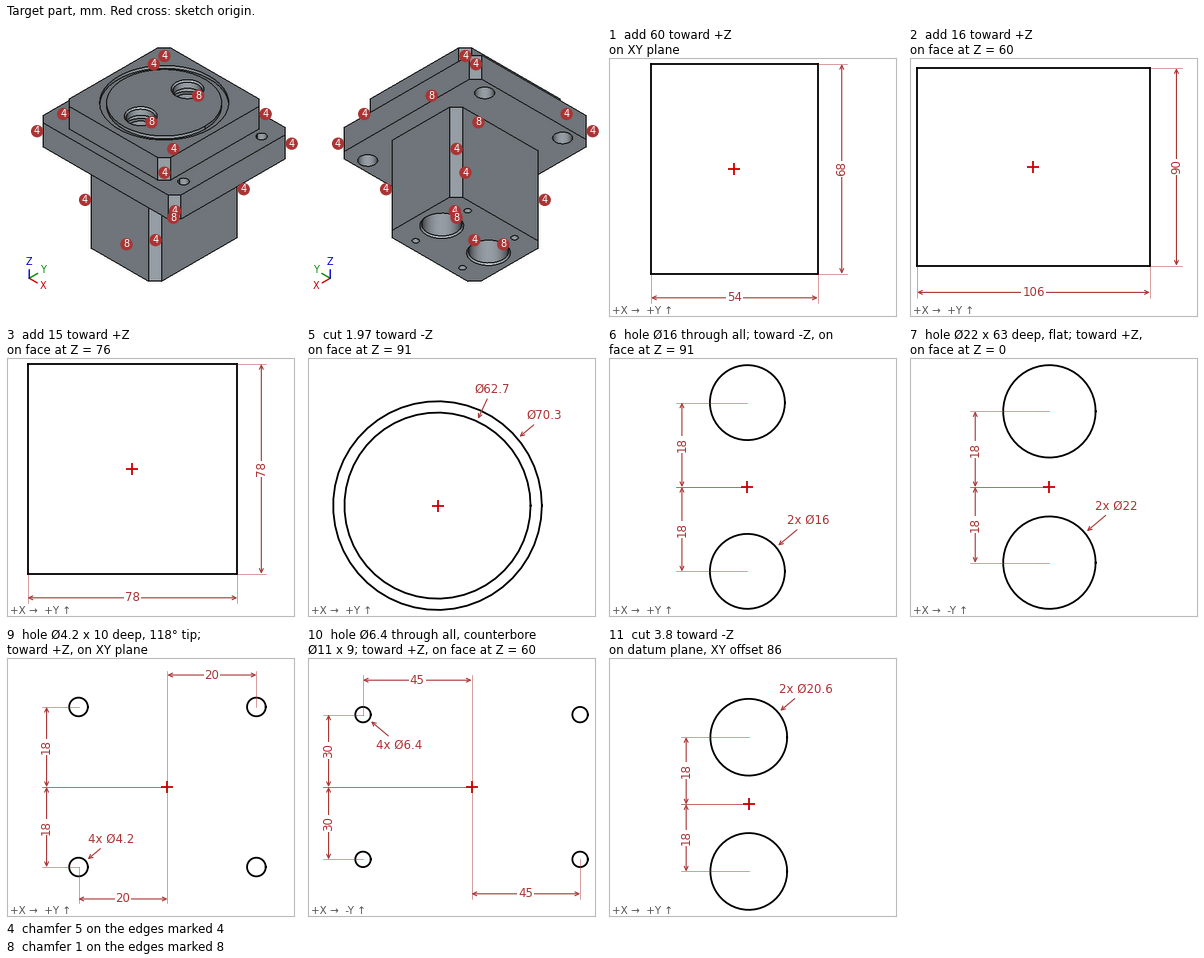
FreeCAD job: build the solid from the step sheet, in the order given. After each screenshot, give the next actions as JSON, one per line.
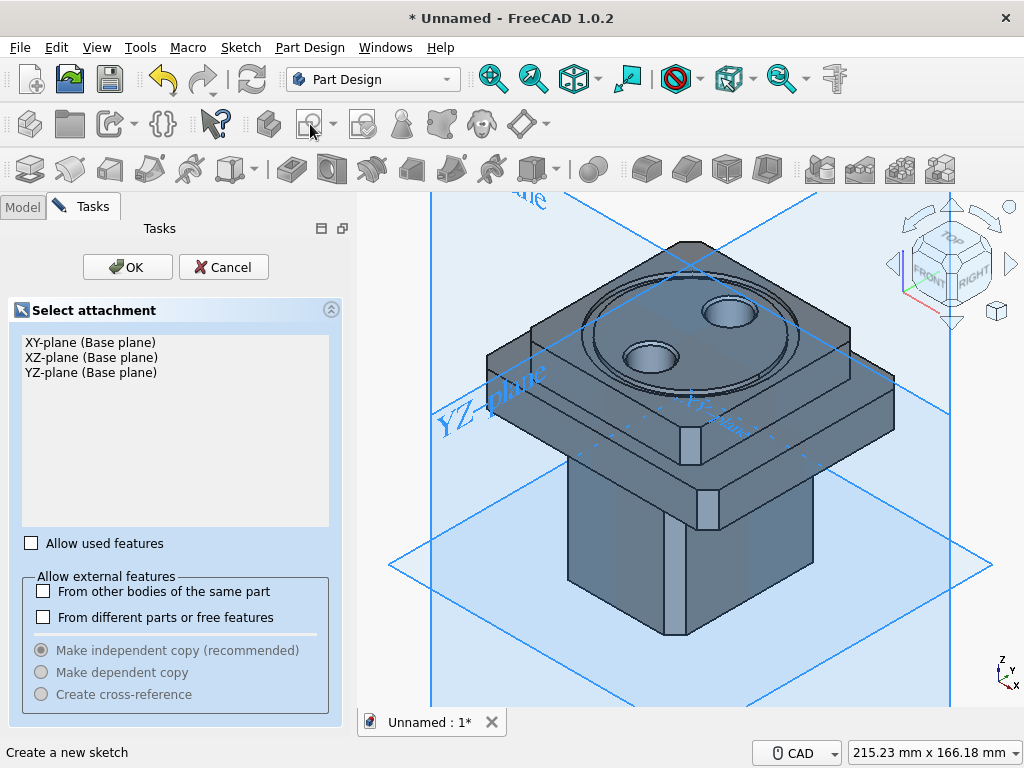
{"action": "left_click", "coordinate": [82, 342]}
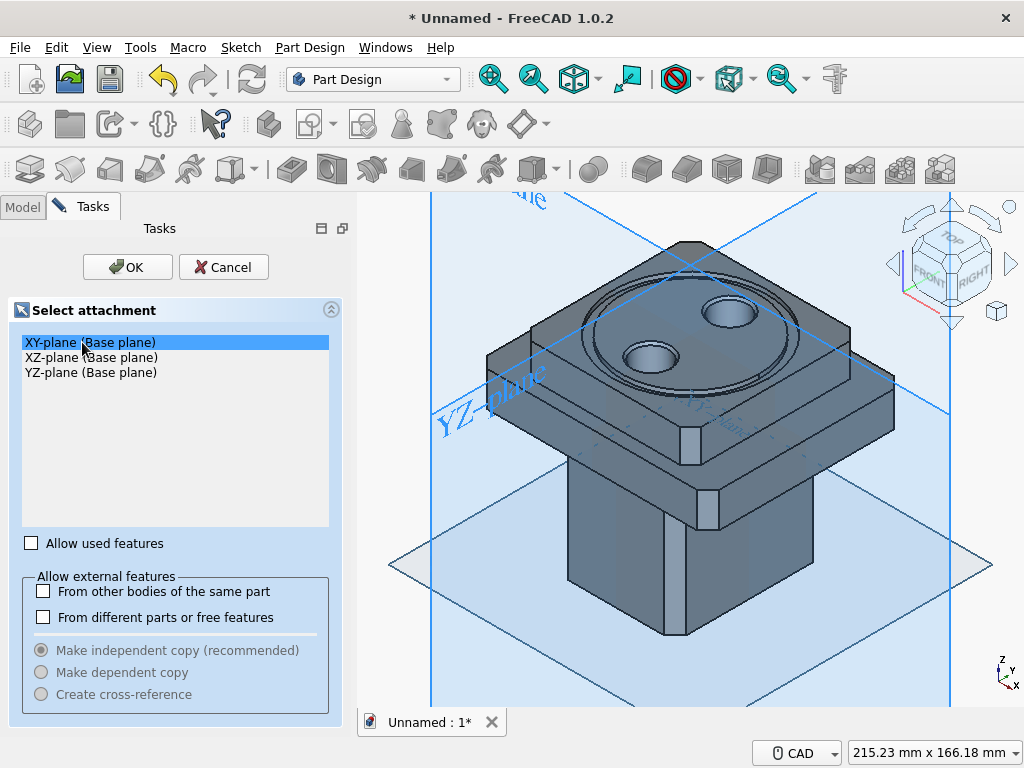
{"action": "left_click", "coordinate": [128, 267]}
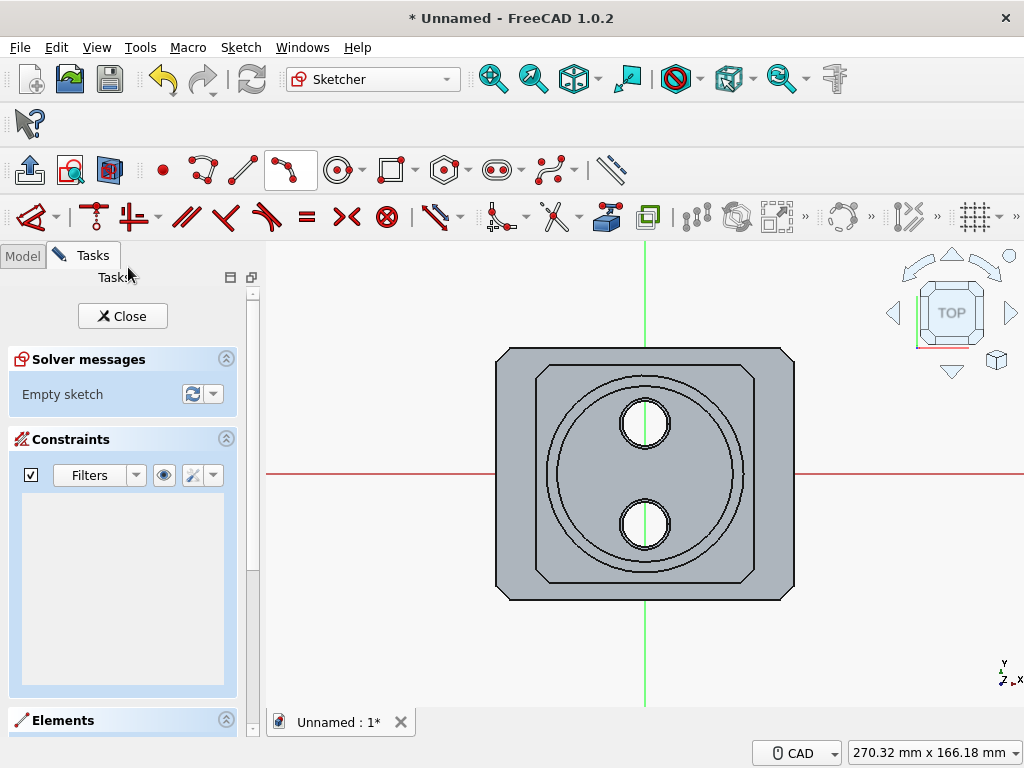
{"action": "key", "text": "q s"}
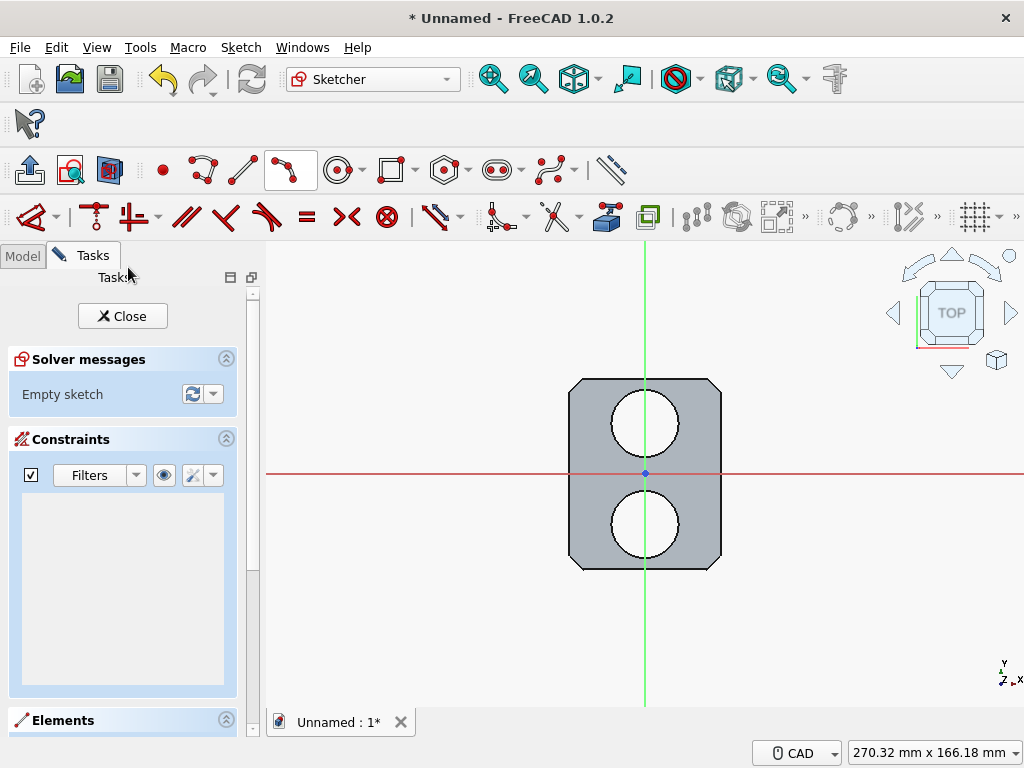
{"action": "scroll", "coordinate": [685, 474], "scroll_direction": "up", "scroll_amount": 5}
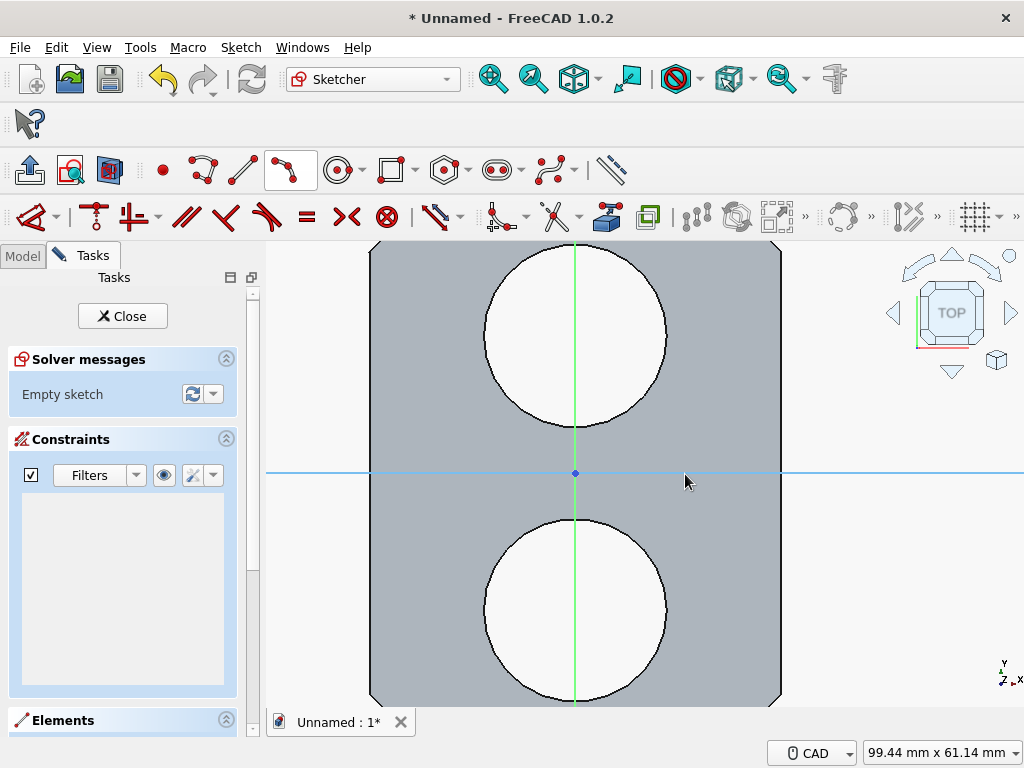
{"action": "left_click", "coordinate": [338, 170]}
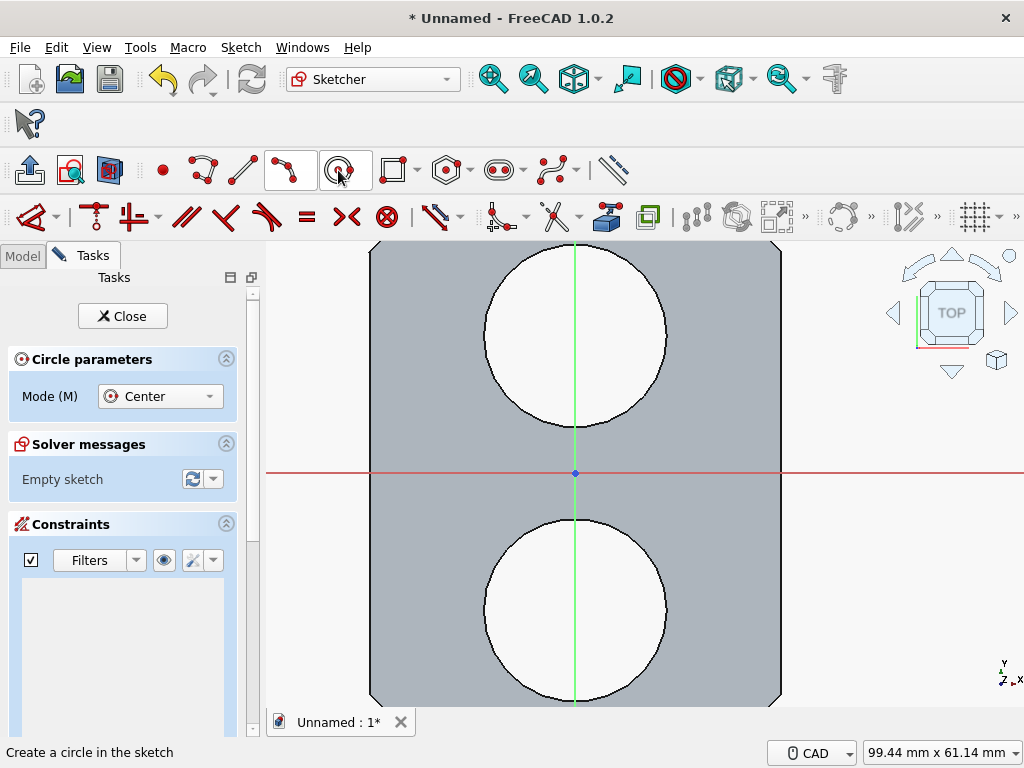
{"action": "scroll", "coordinate": [423, 610], "scroll_direction": "up", "scroll_amount": 2}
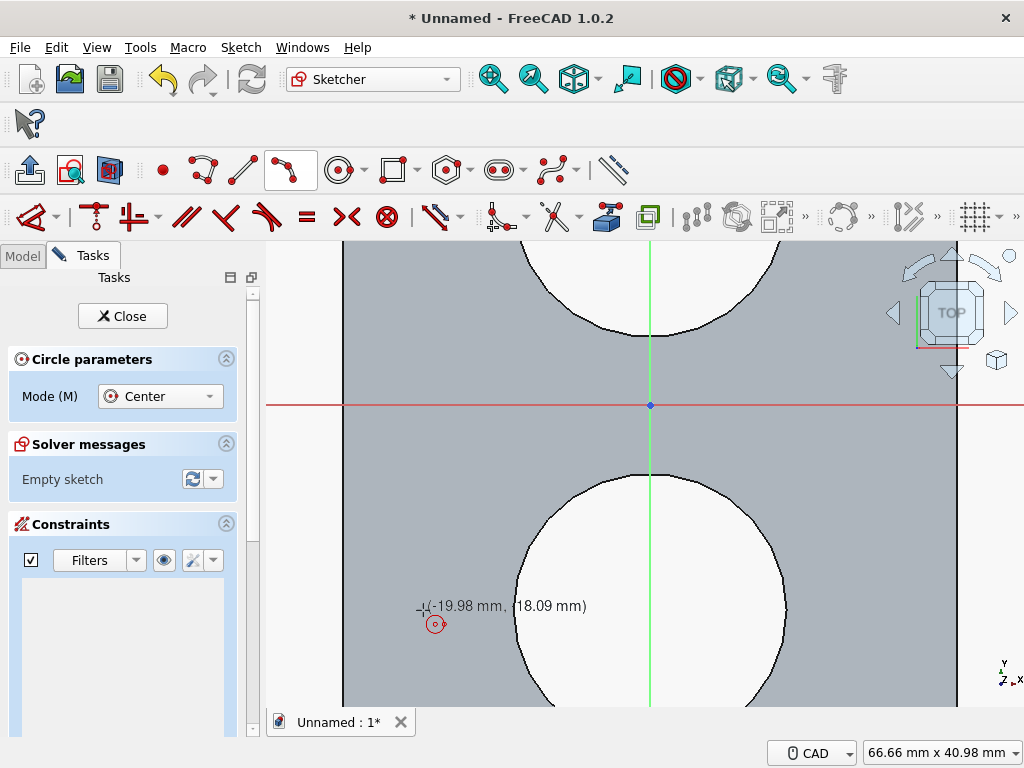
{"action": "left_click", "coordinate": [423, 610]}
{"action": "mouse_move", "coordinate": [440, 593]}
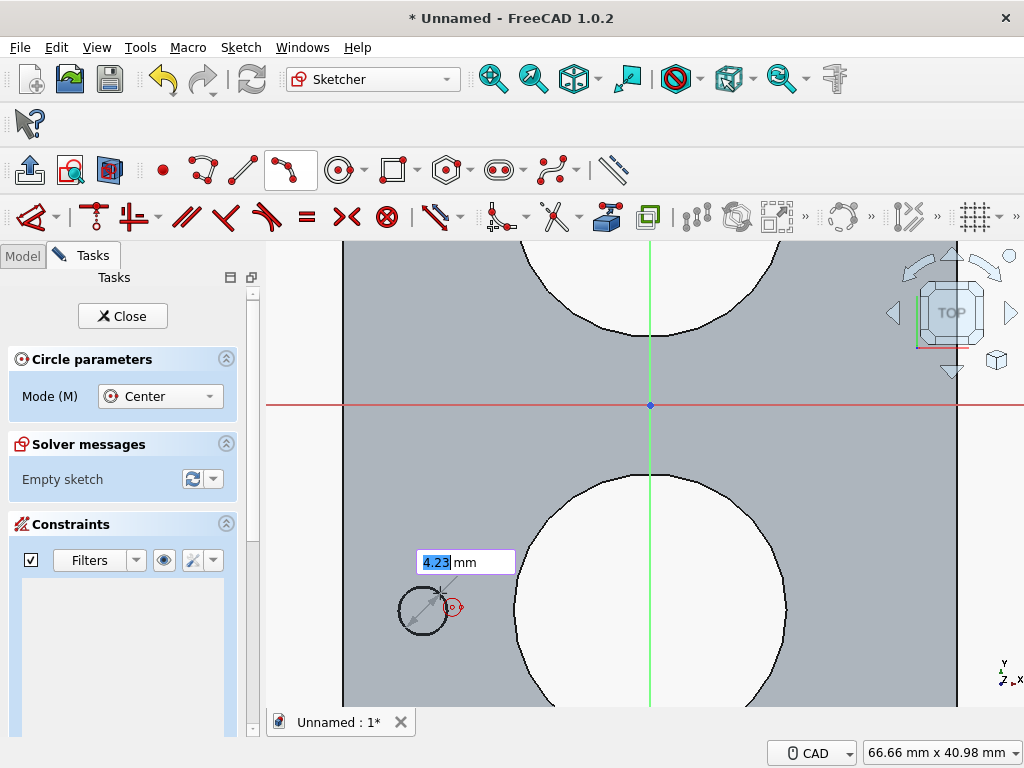
{"action": "type", "text": "4.2"}
{"action": "key", "text": "Return"}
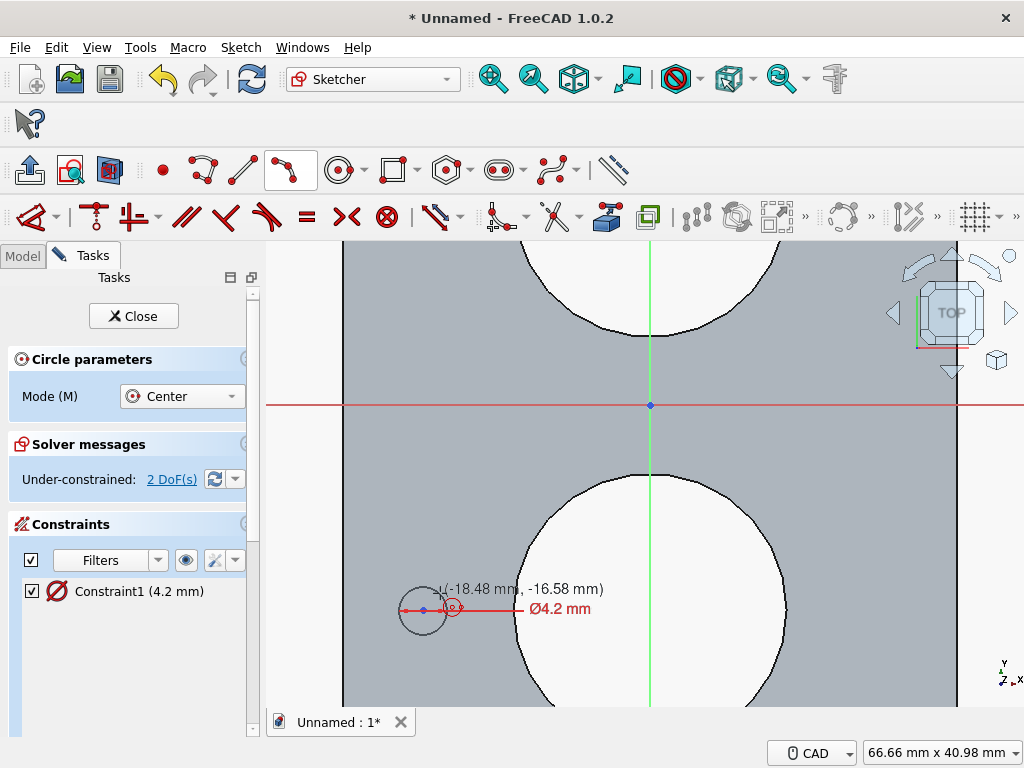
{"action": "scroll", "coordinate": [427, 613], "scroll_direction": "down", "scroll_amount": 2}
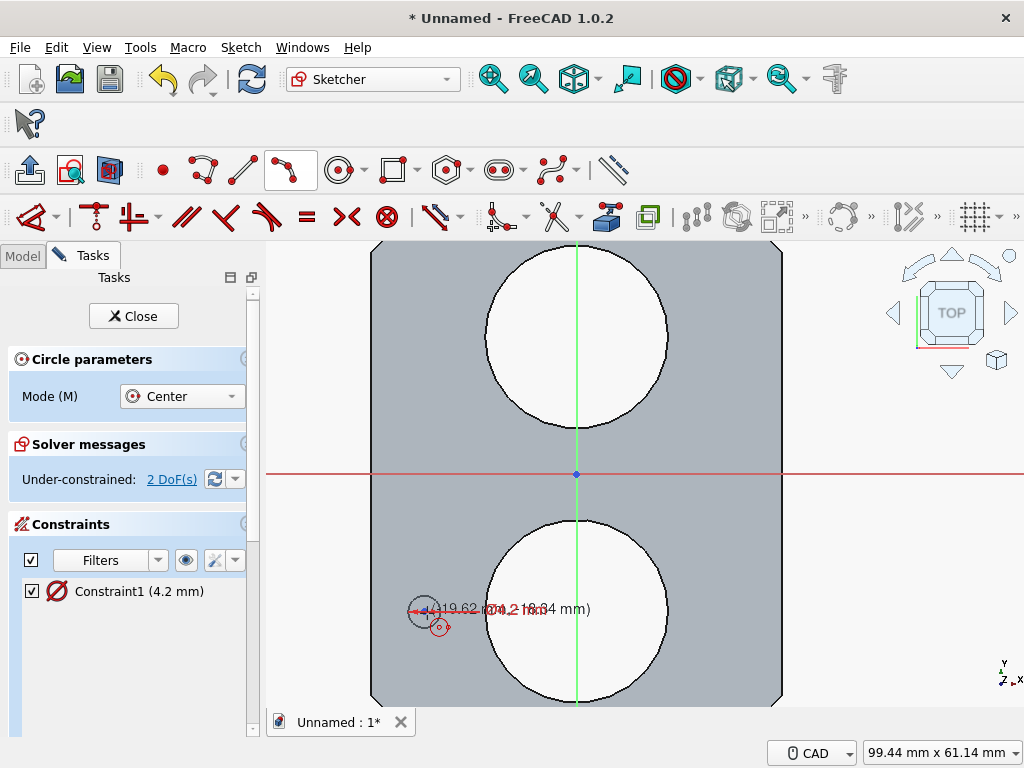
{"action": "scroll", "coordinate": [424, 337], "scroll_direction": "up", "scroll_amount": 2}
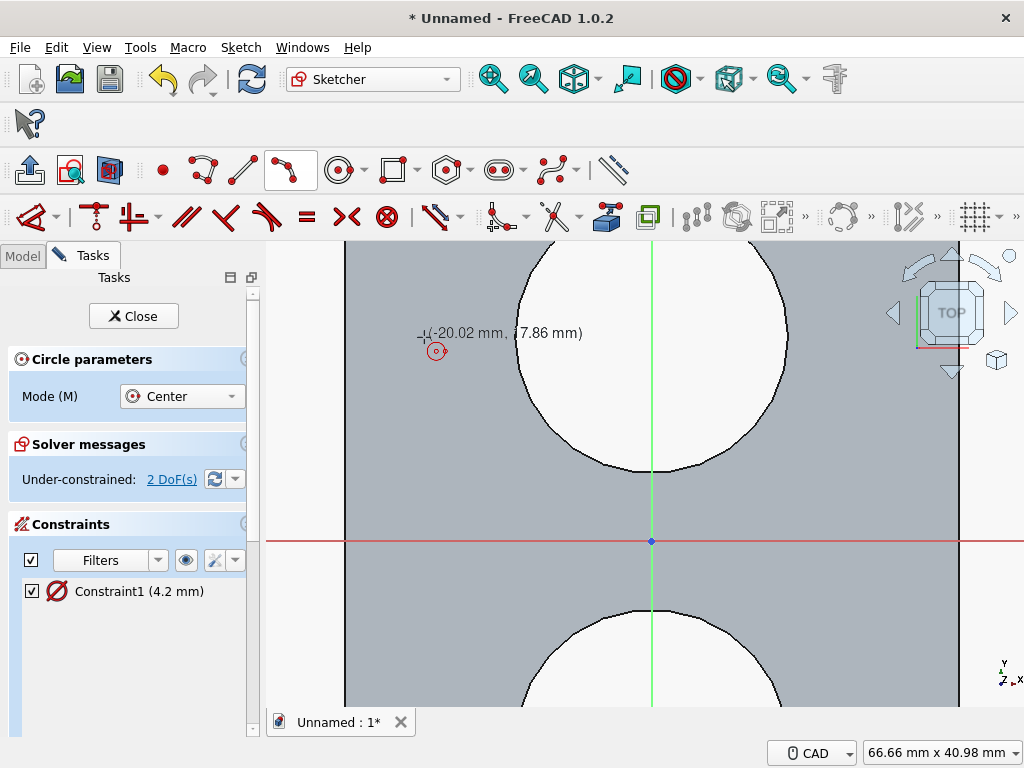
{"action": "left_click", "coordinate": [424, 337]}
{"action": "mouse_move", "coordinate": [441, 320]}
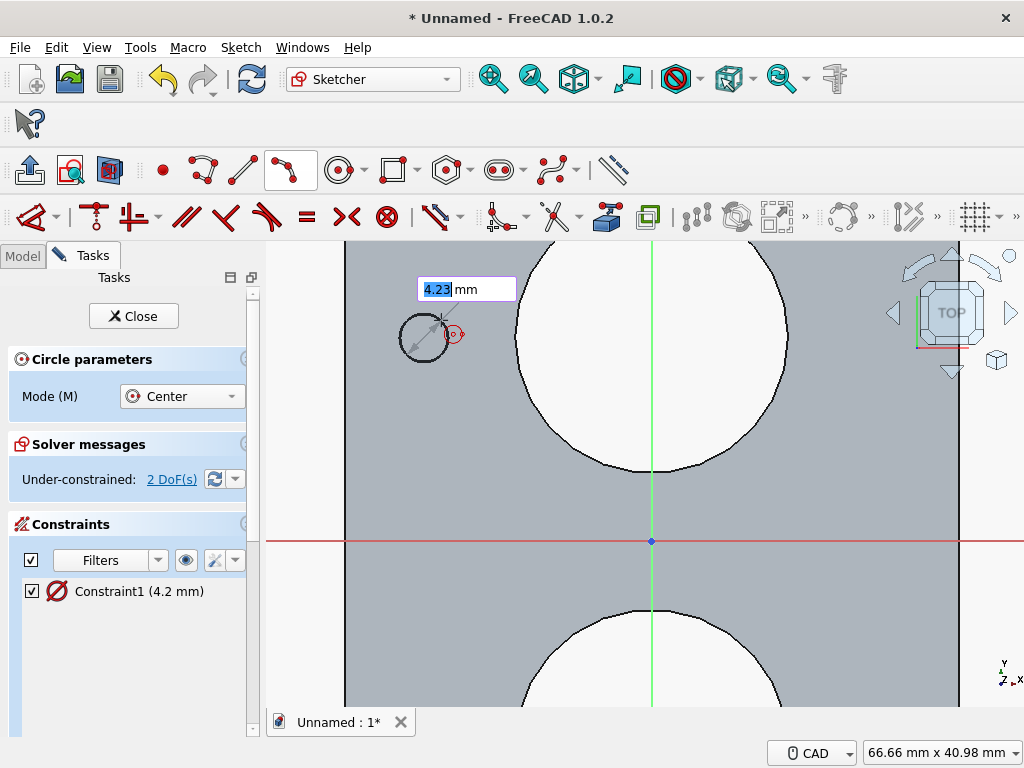
{"action": "type", "text": "4.2"}
{"action": "key", "text": "Return"}